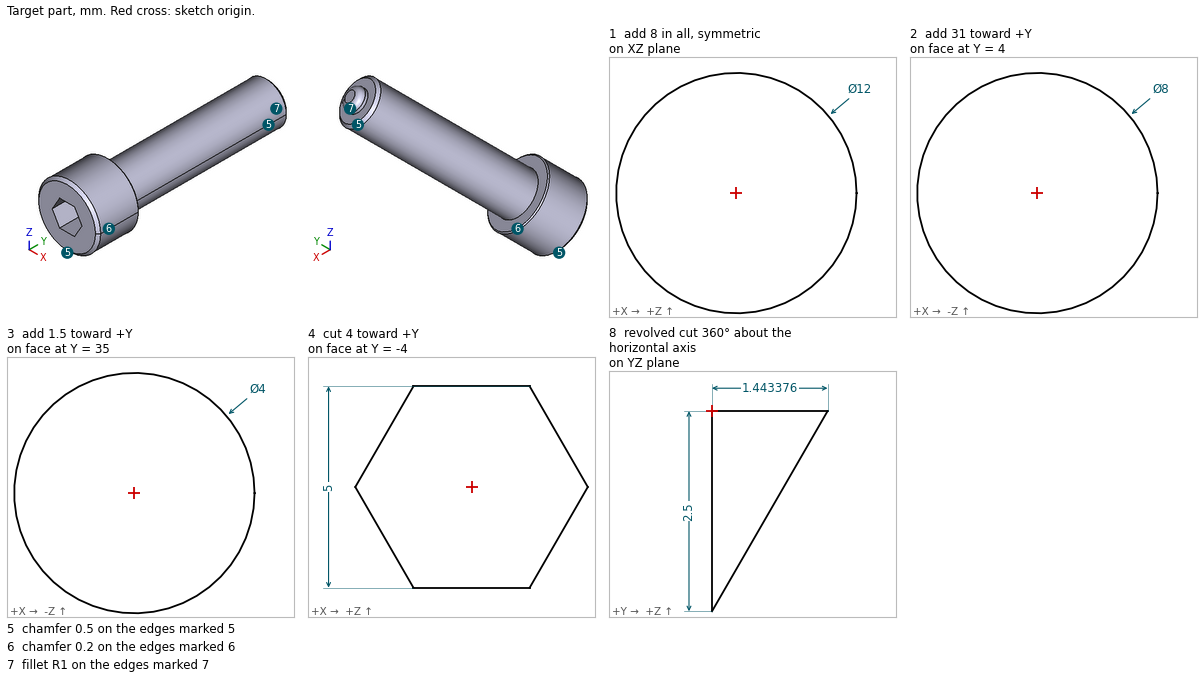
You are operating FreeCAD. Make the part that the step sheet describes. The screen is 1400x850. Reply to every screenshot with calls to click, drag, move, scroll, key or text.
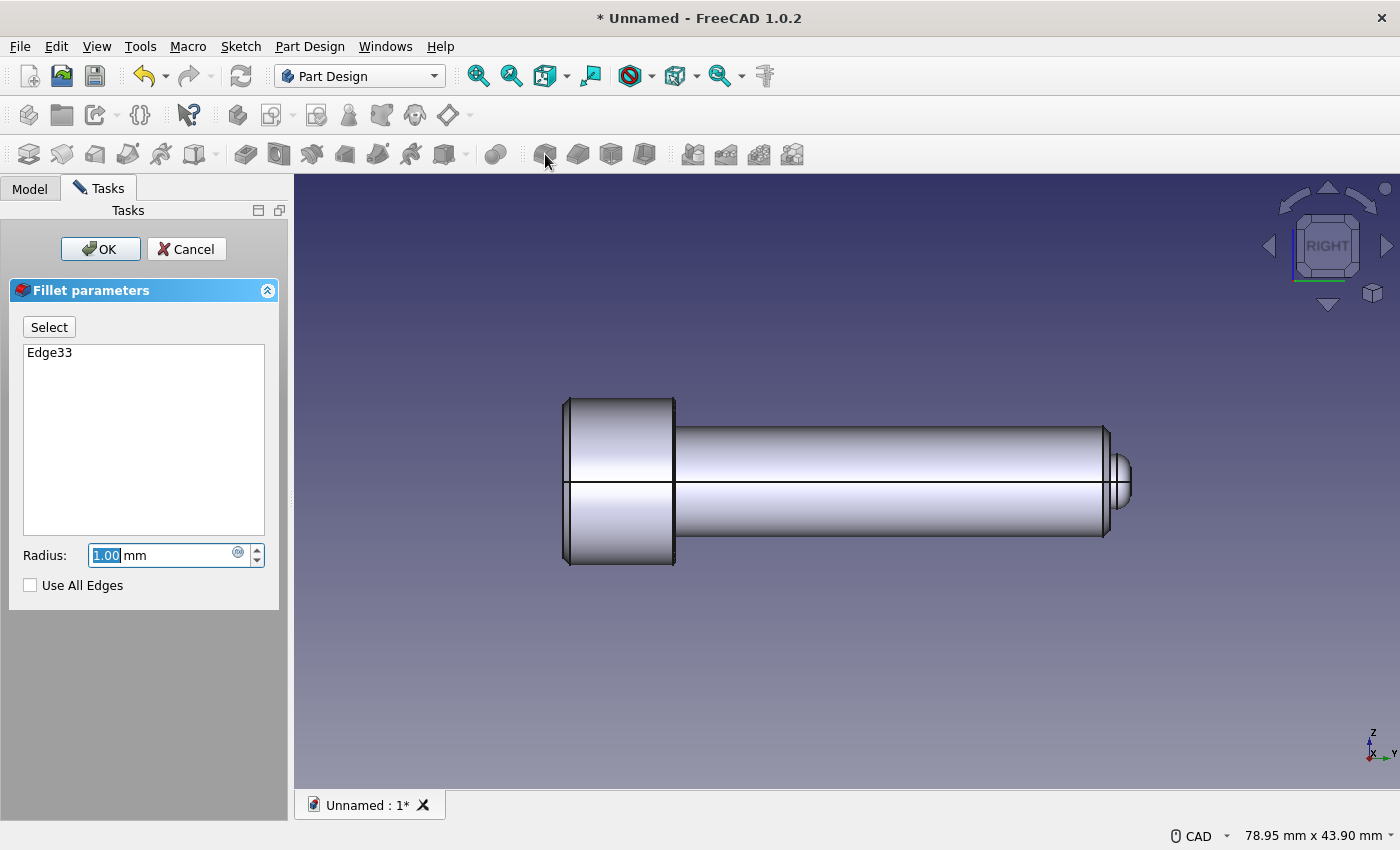
text(1)
key(Tab)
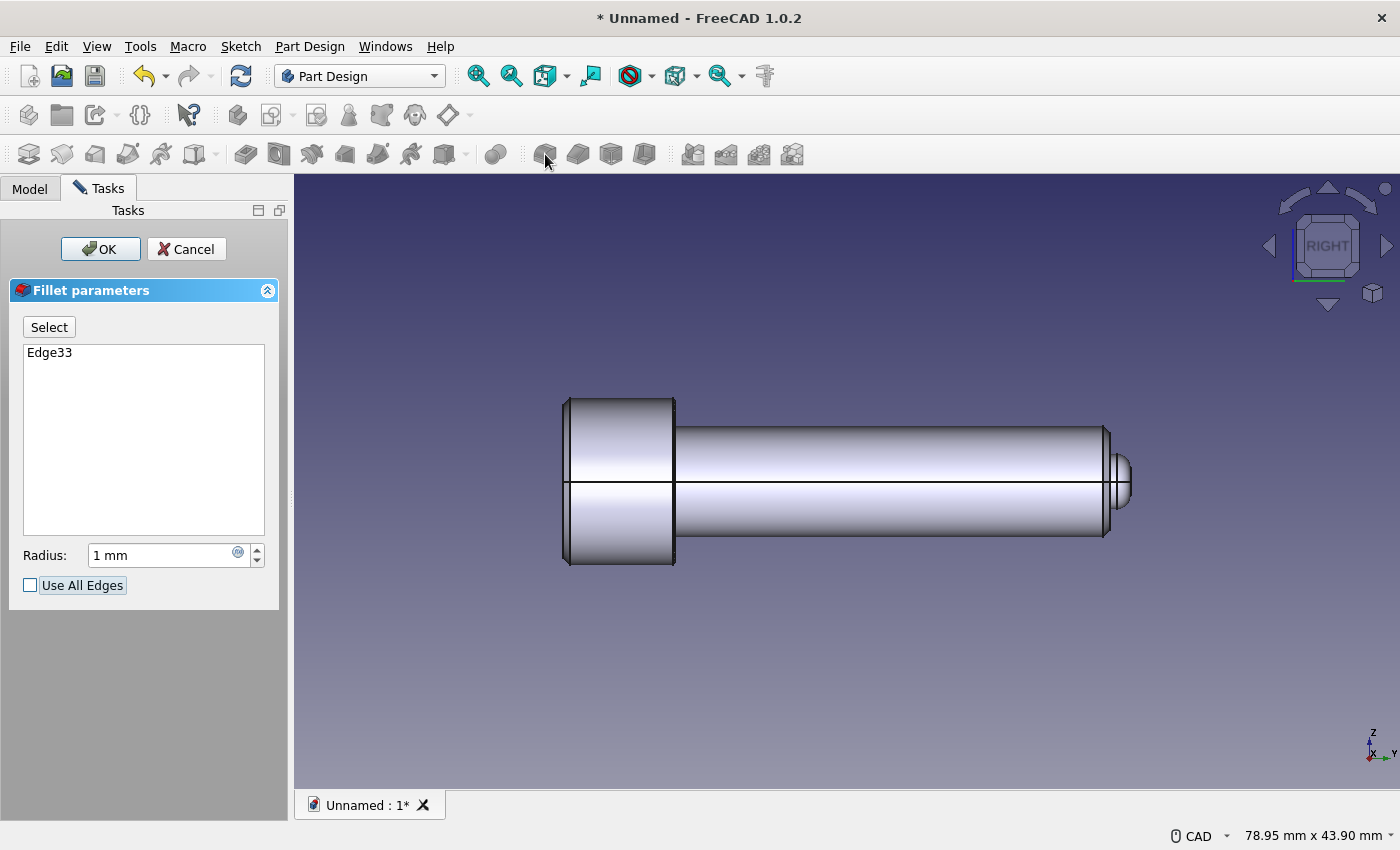
click(101, 249)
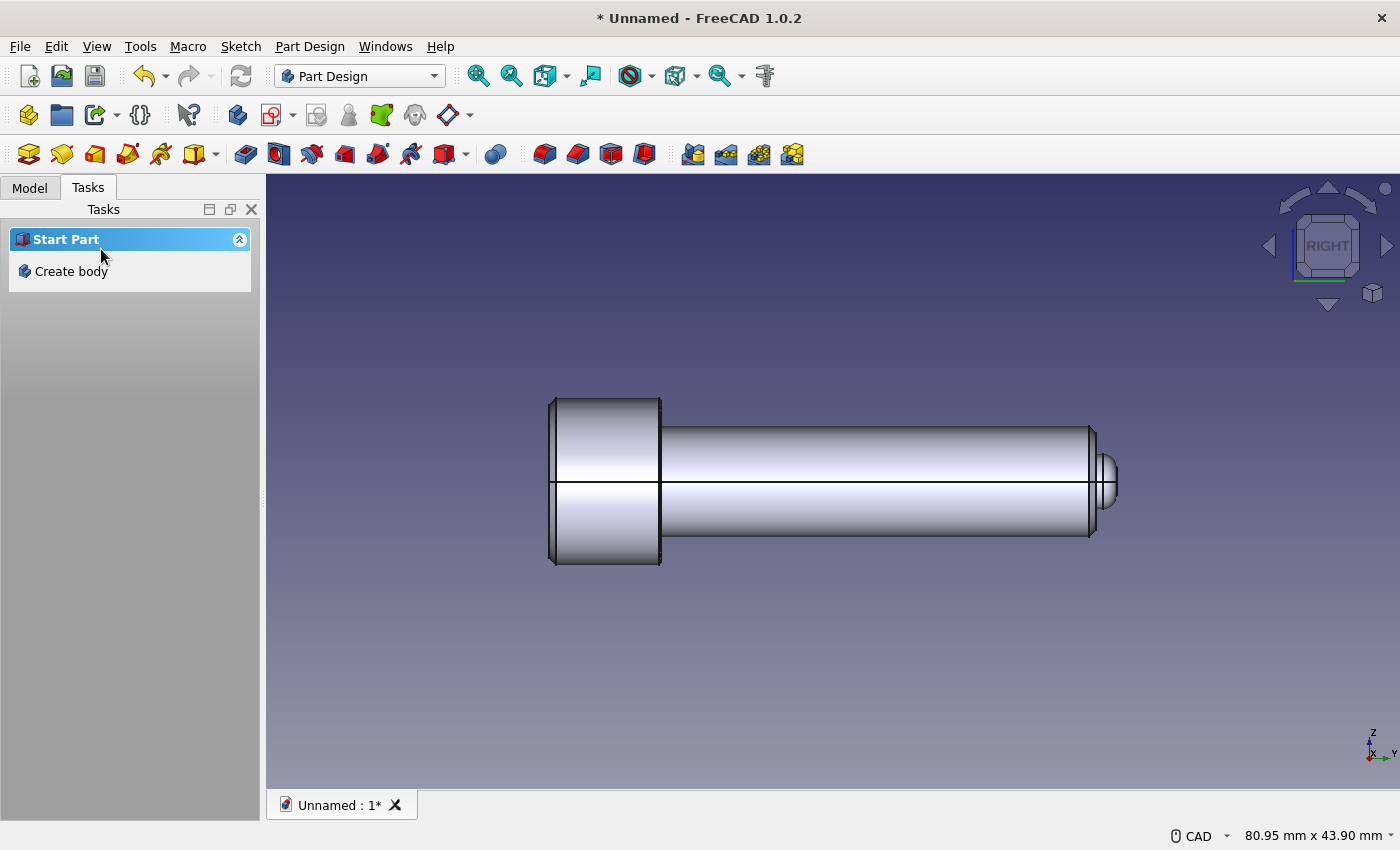
click(270, 116)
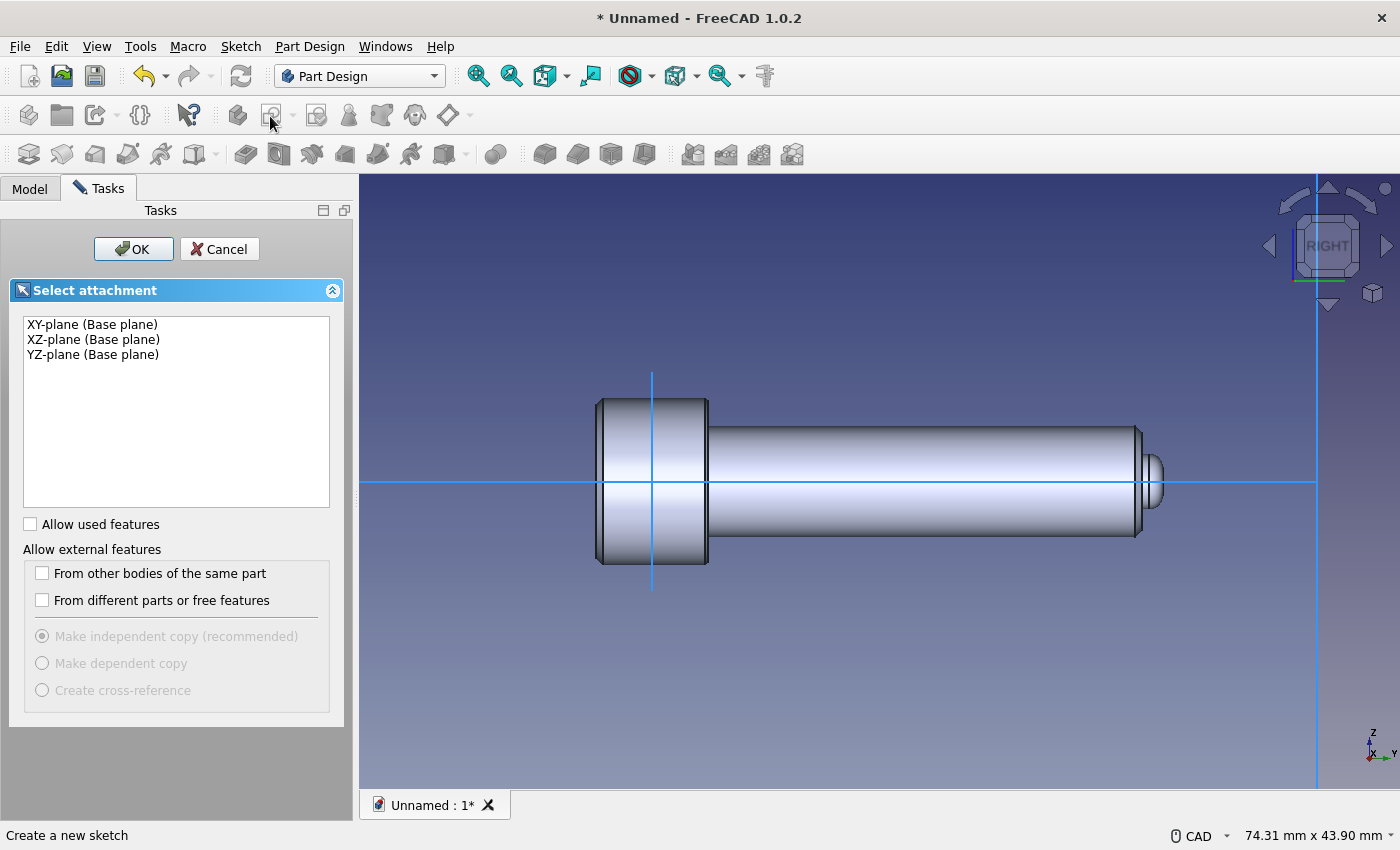
click(84, 354)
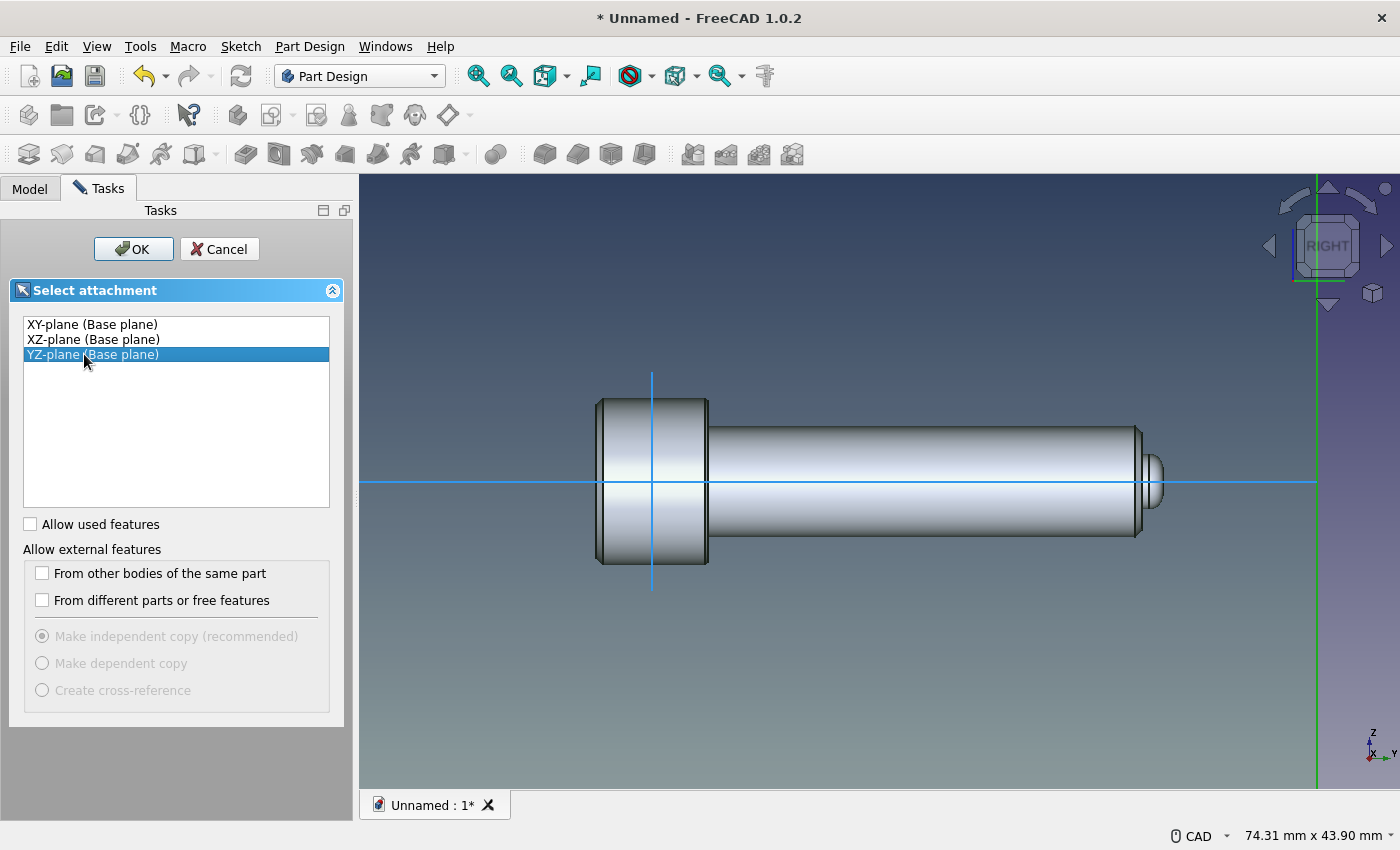
click(134, 249)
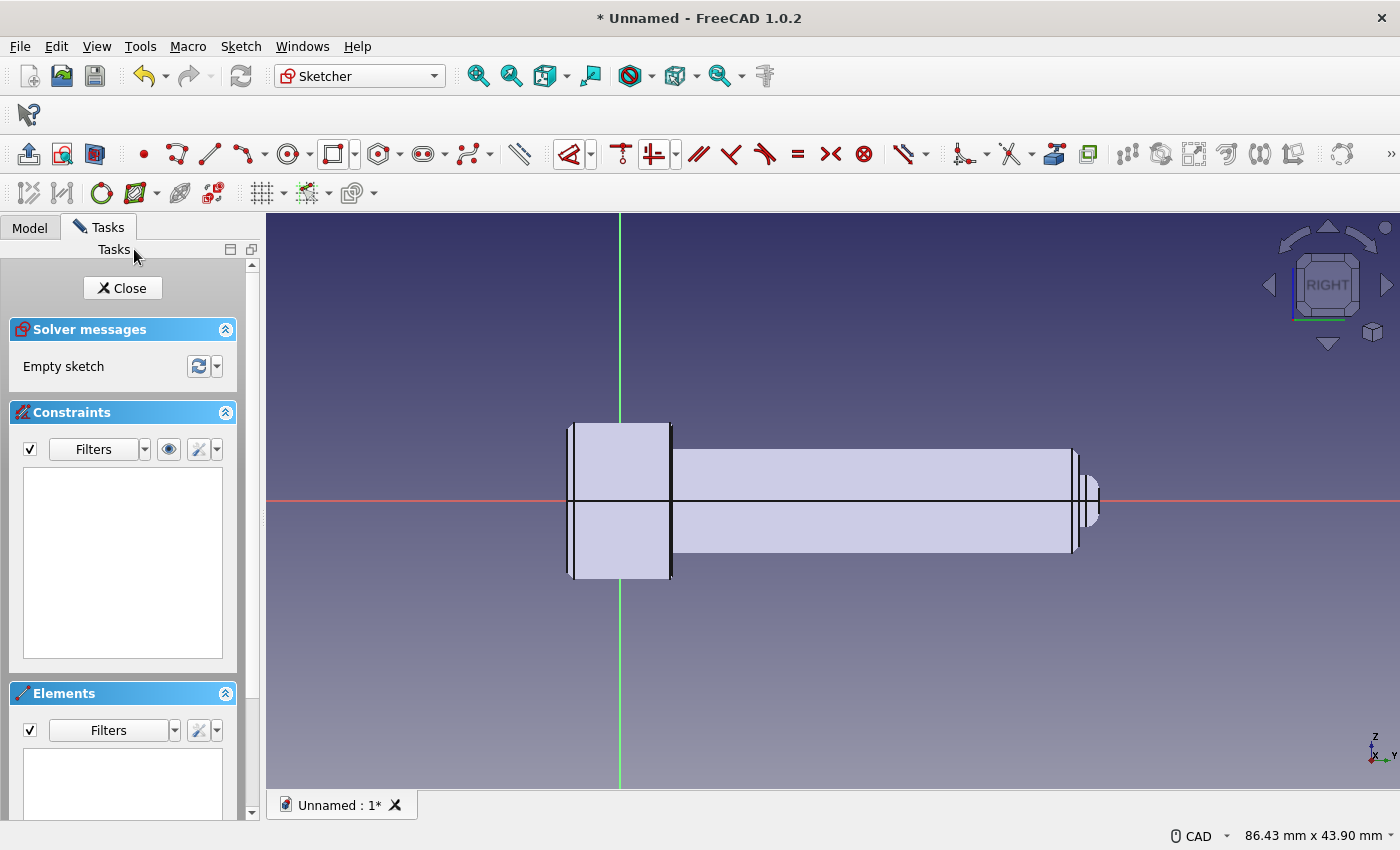
click(95, 154)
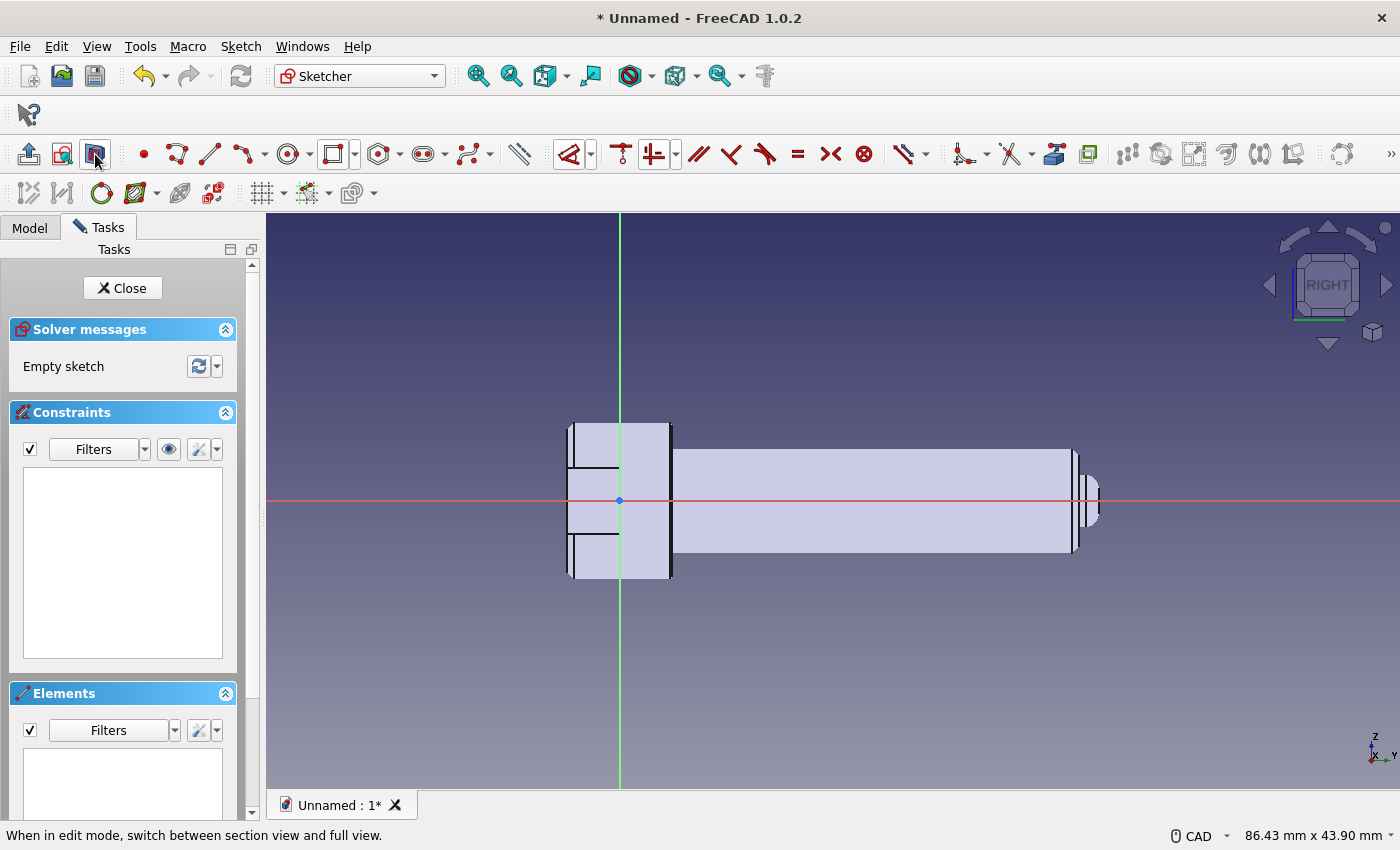
scroll(616, 519, up, 12)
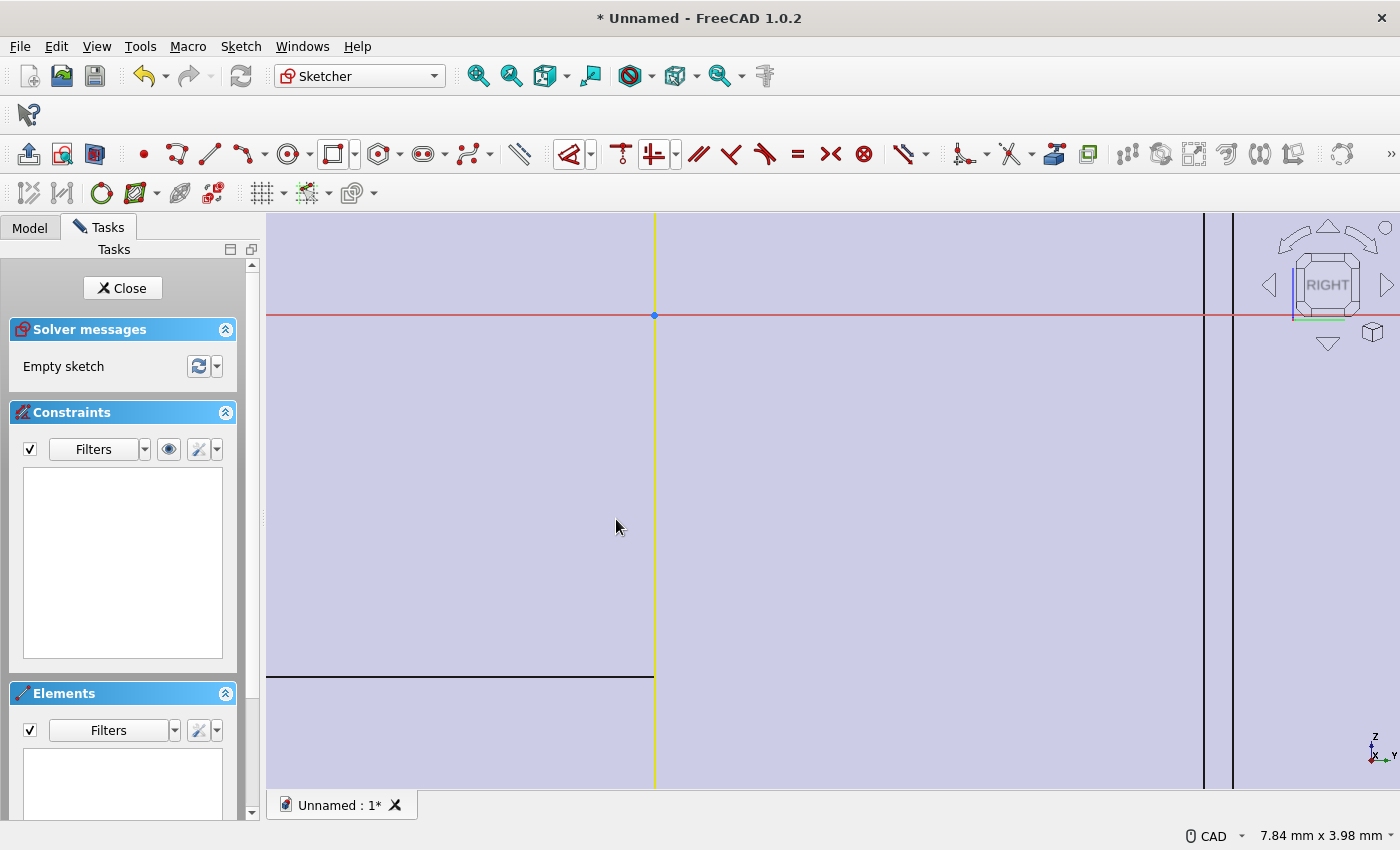
click(177, 154)